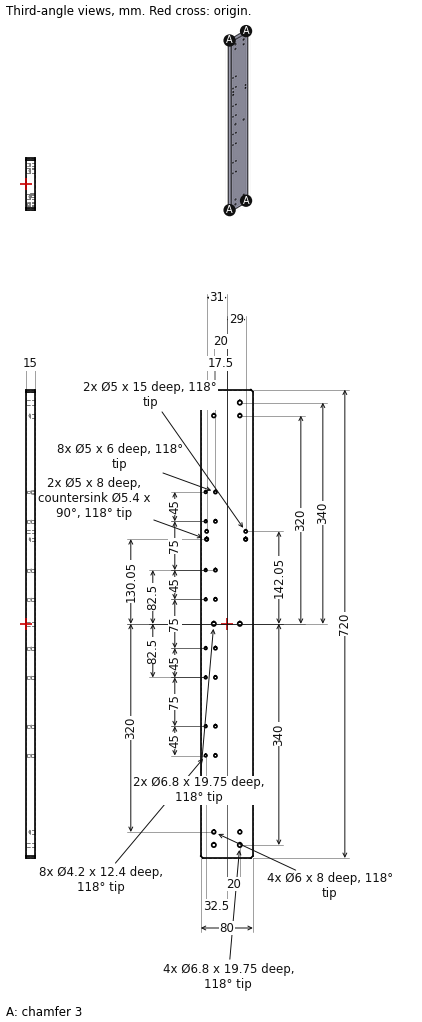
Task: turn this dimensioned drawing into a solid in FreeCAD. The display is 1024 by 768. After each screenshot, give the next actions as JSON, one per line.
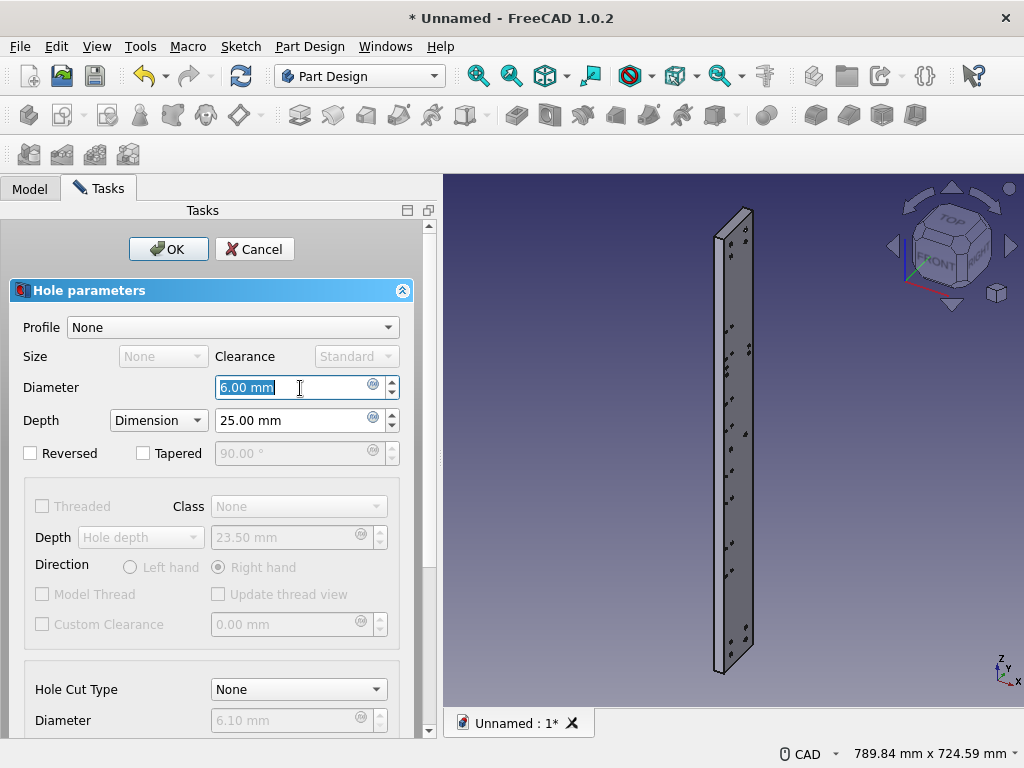
{"action": "type", "text": "5"}
{"action": "key", "text": "Tab"}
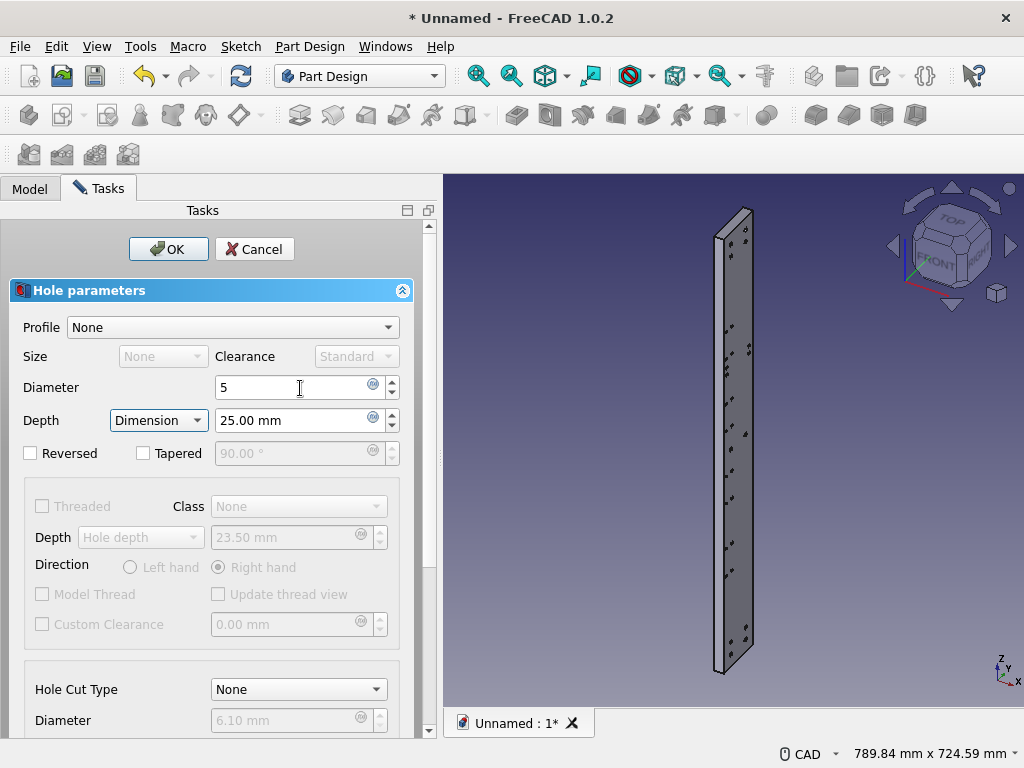
{"action": "triple_click", "coordinate": [300, 420]}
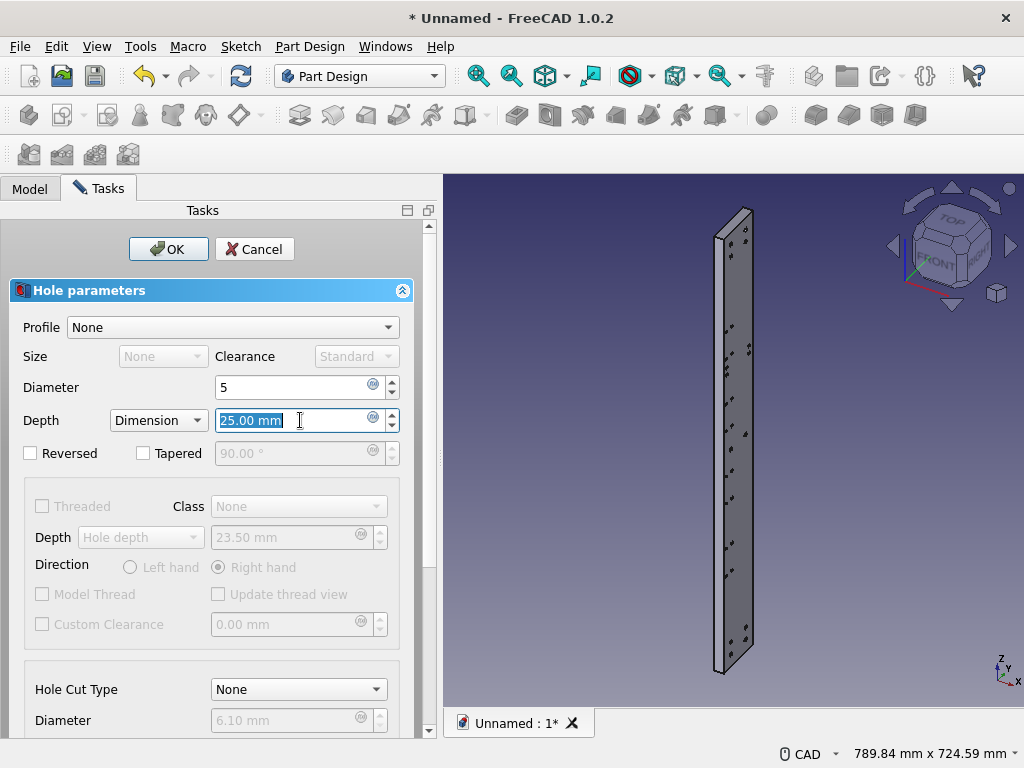
{"action": "type", "text": "8"}
{"action": "key", "text": "Tab"}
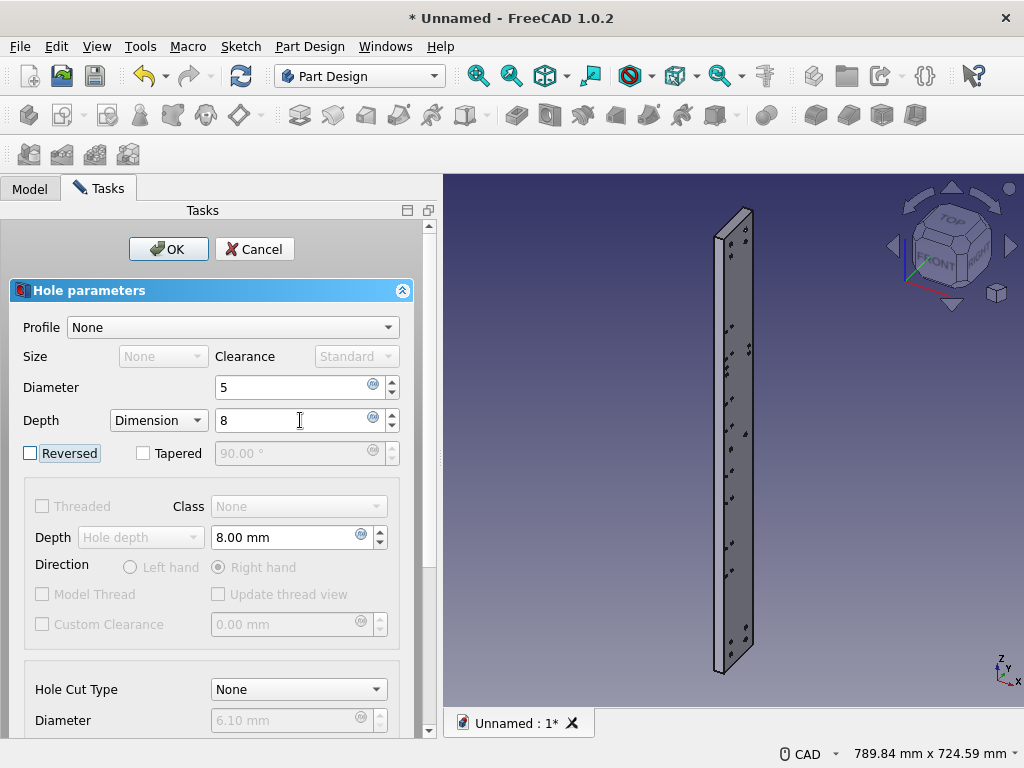
{"action": "left_click", "coordinate": [300, 690]}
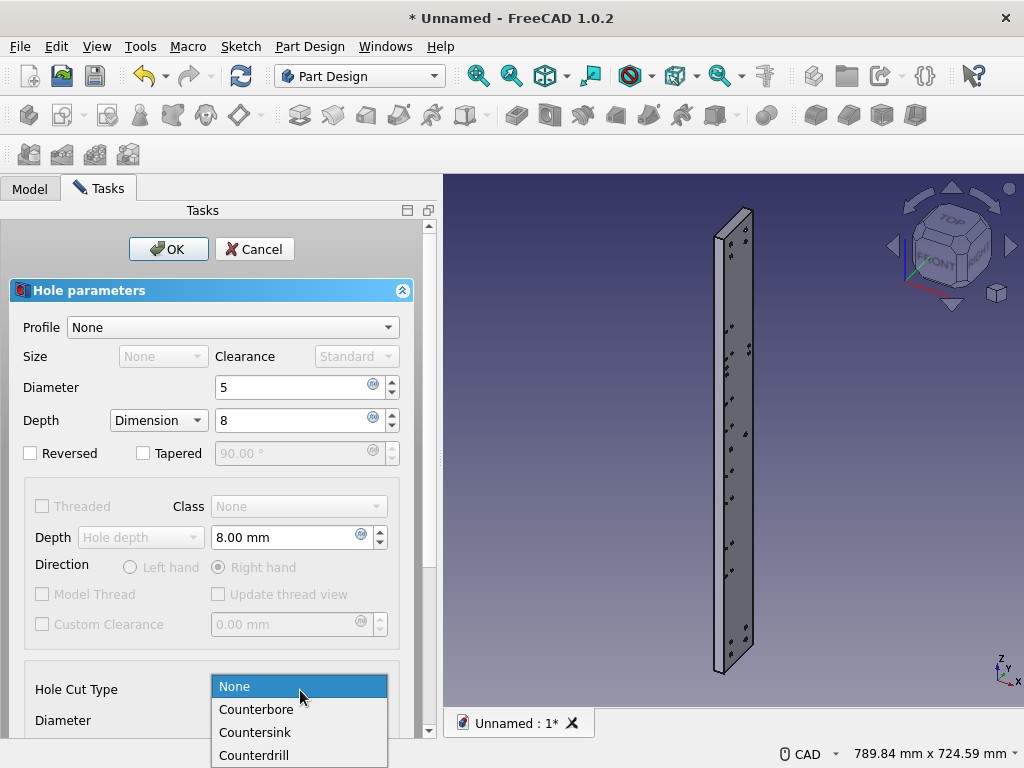
{"action": "left_click", "coordinate": [298, 732]}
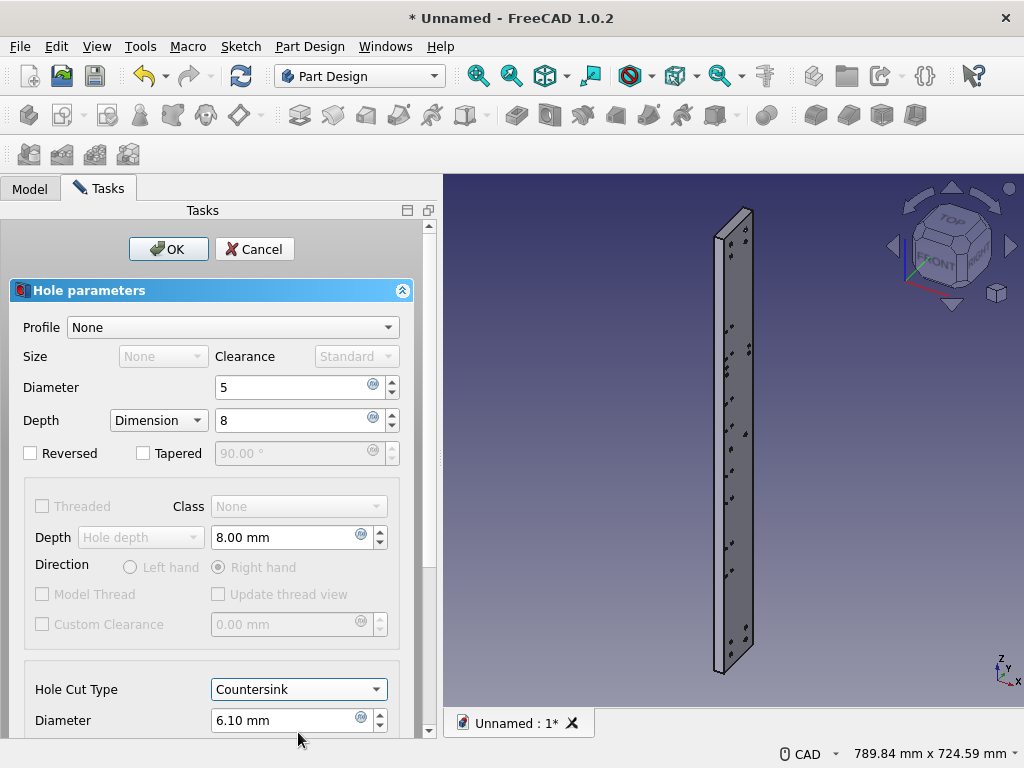
{"action": "triple_click", "coordinate": [292, 720]}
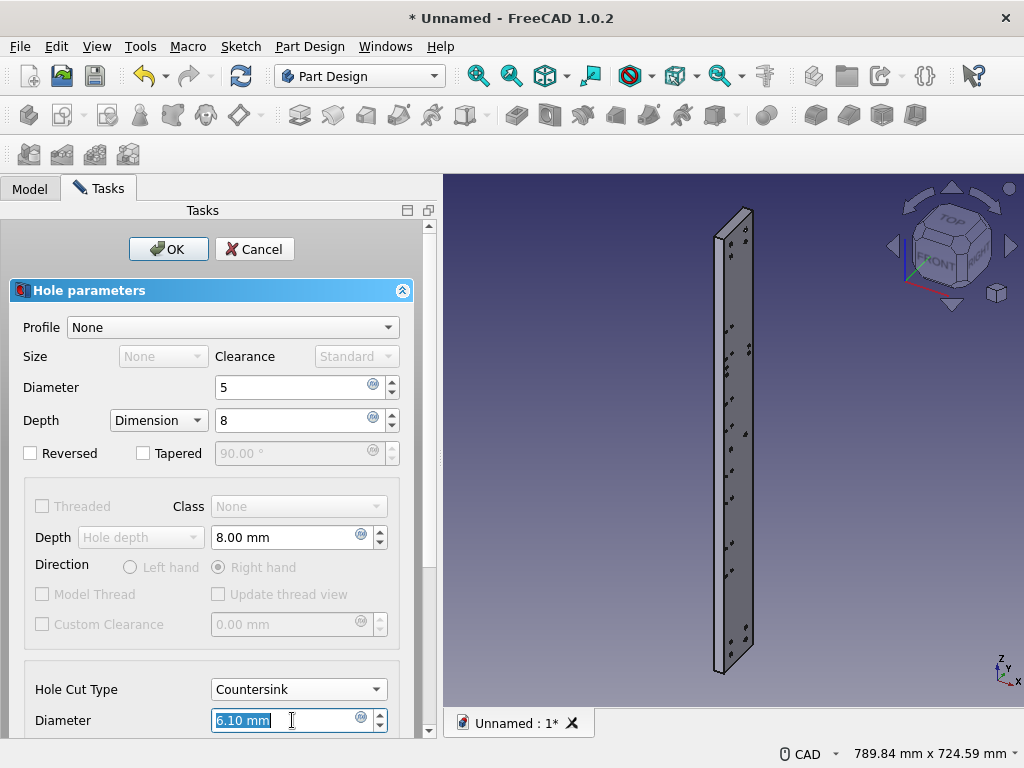
{"action": "type", "text": "5.4"}
{"action": "key", "text": "Tab"}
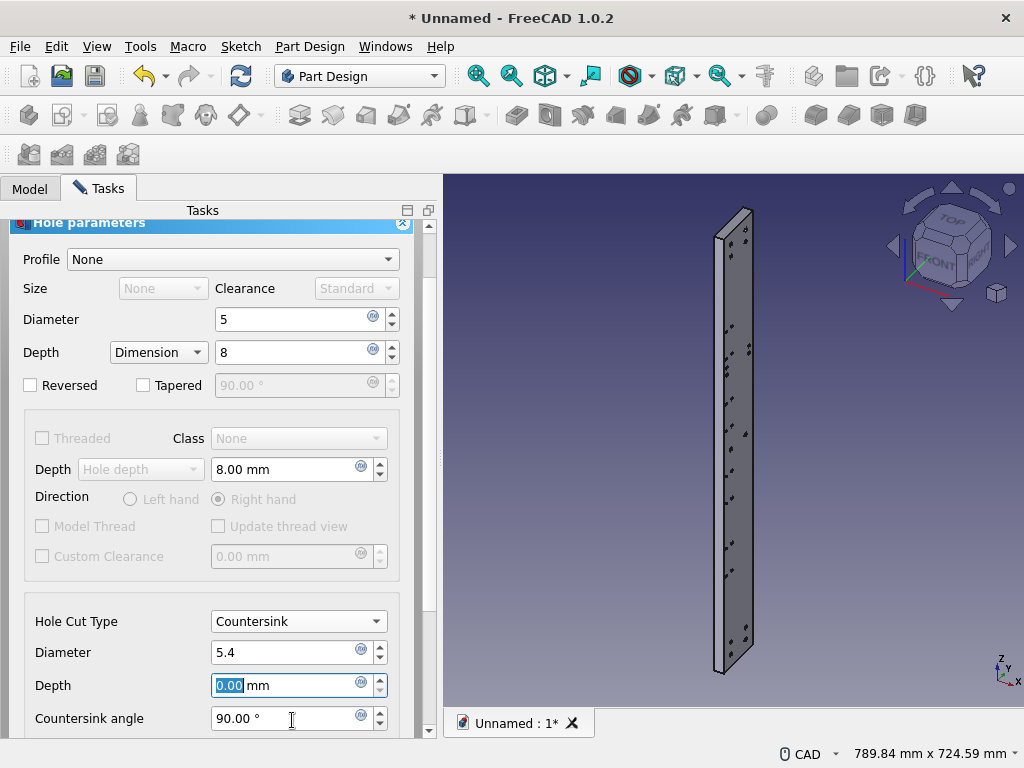
{"action": "scroll", "coordinate": [429, 479], "scroll_direction": "up", "scroll_amount": 2}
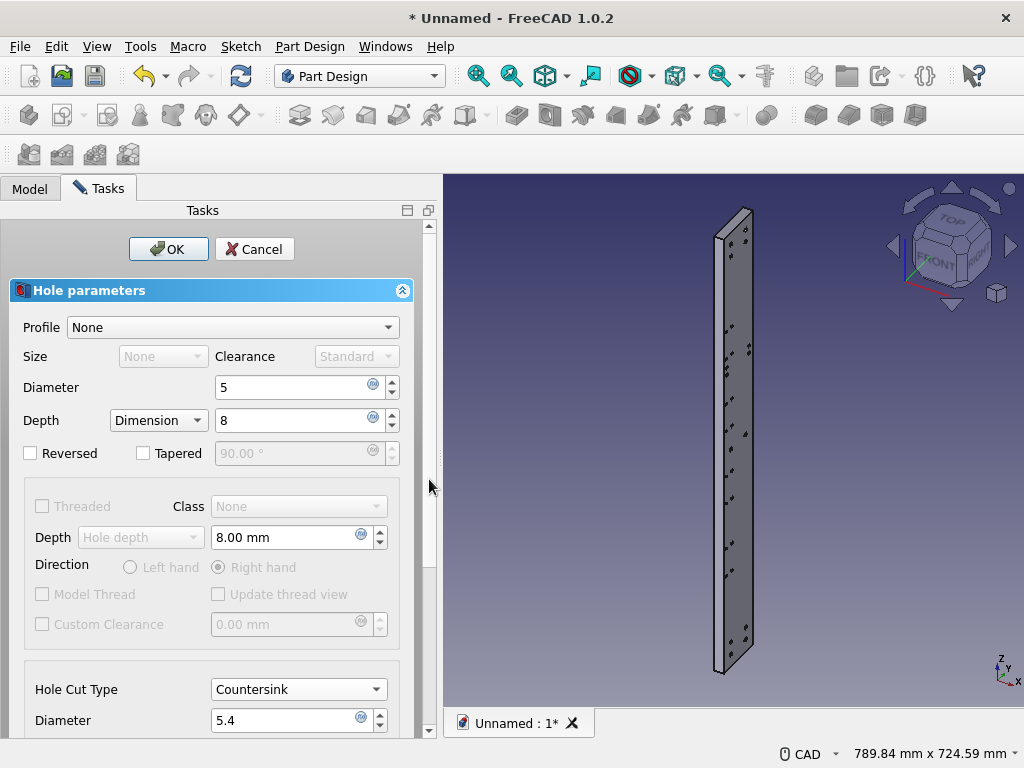
{"action": "left_click", "coordinate": [169, 249]}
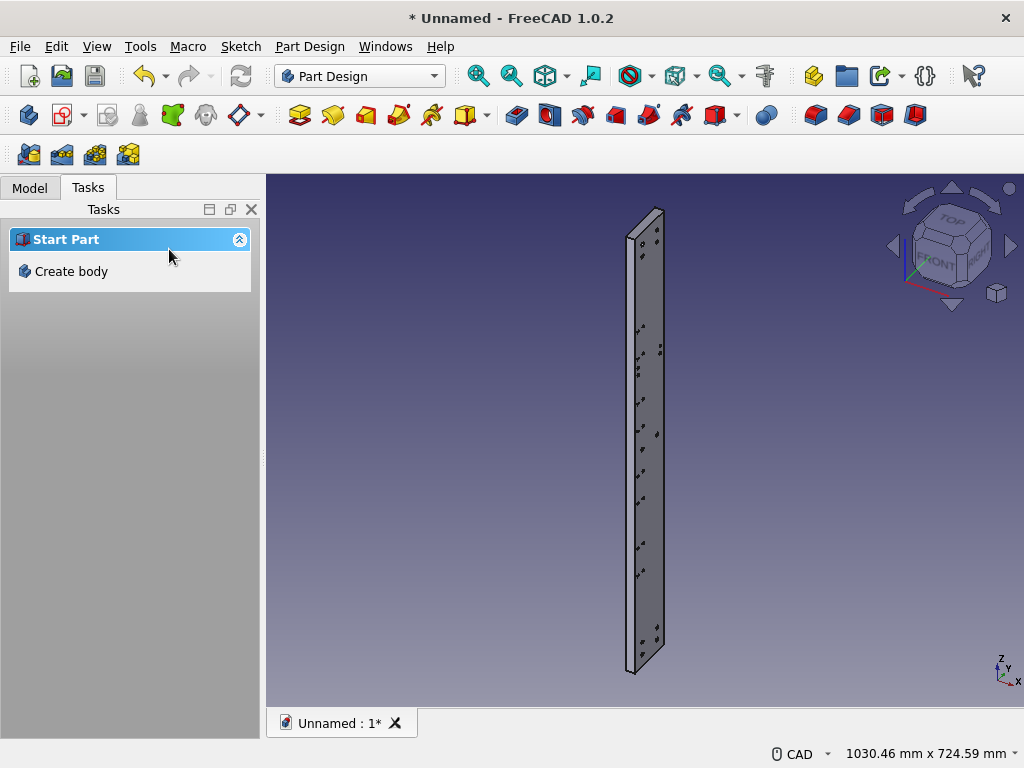
{"action": "left_click", "coordinate": [629, 237]}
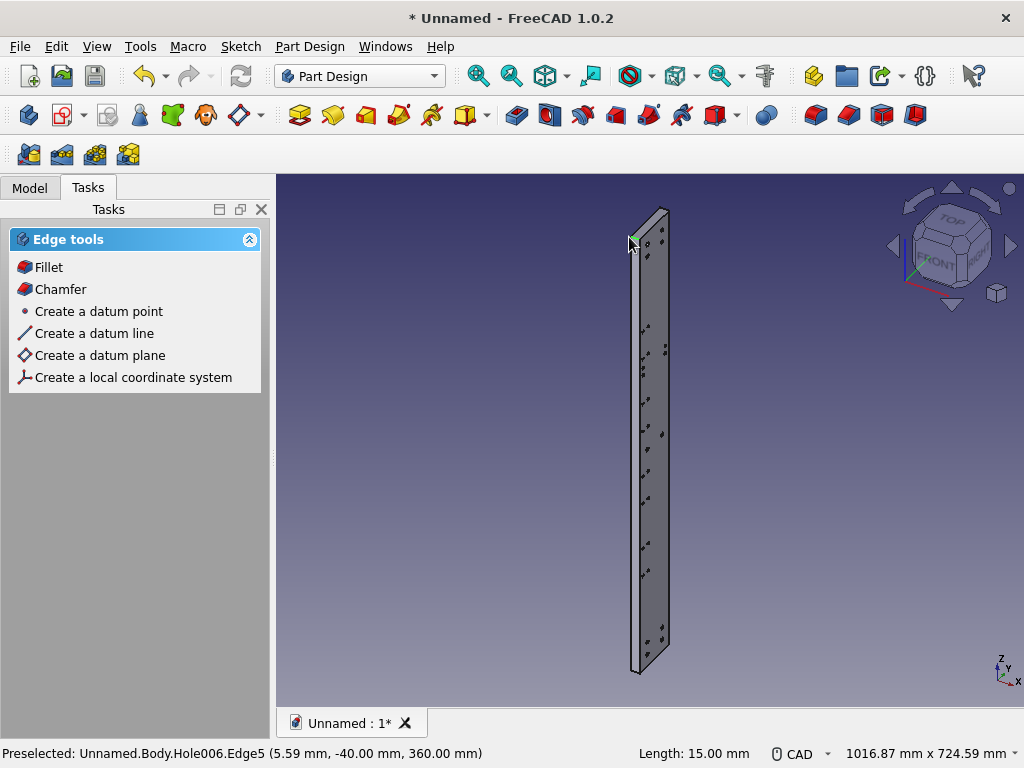
{"action": "scroll", "coordinate": [635, 671], "scroll_direction": "up", "scroll_amount": 7}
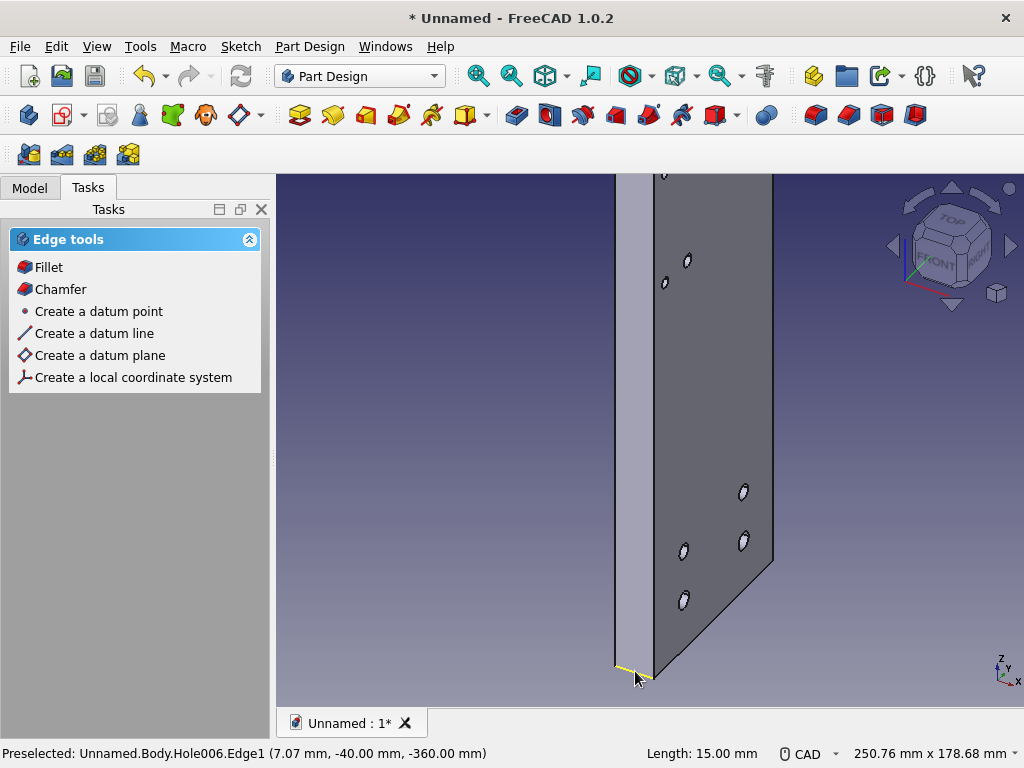
{"action": "key", "text": "v f"}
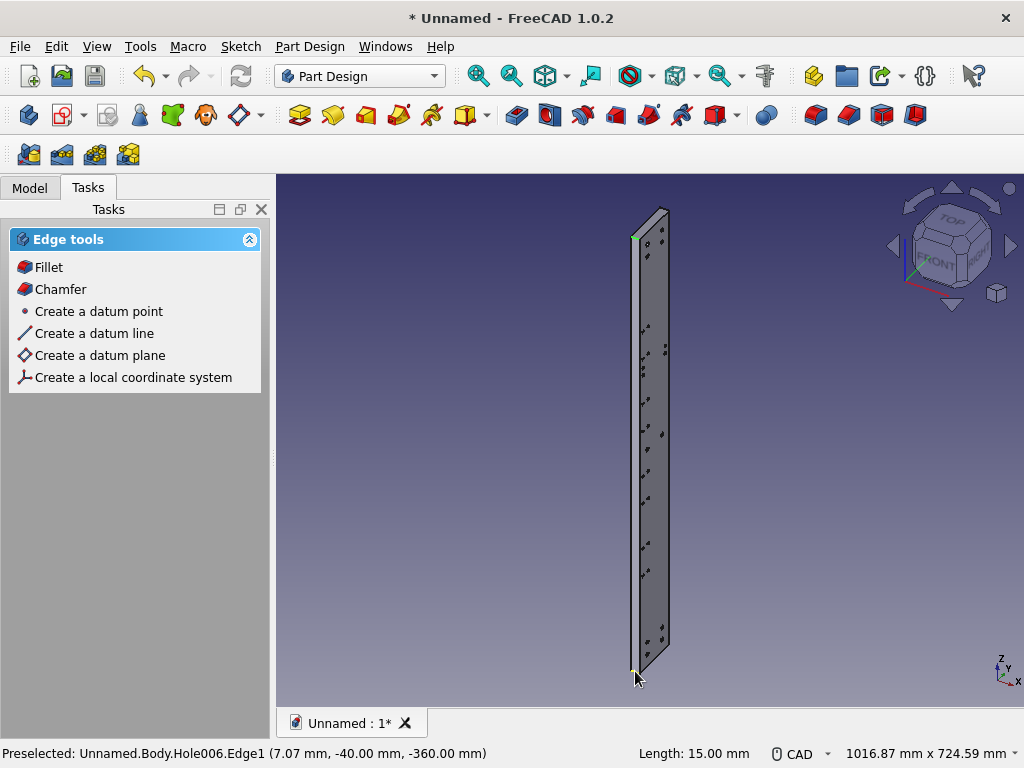
{"action": "key", "text": "0"}